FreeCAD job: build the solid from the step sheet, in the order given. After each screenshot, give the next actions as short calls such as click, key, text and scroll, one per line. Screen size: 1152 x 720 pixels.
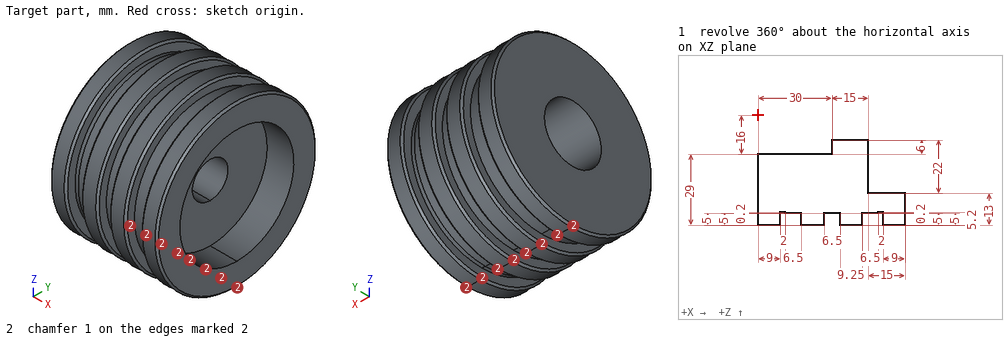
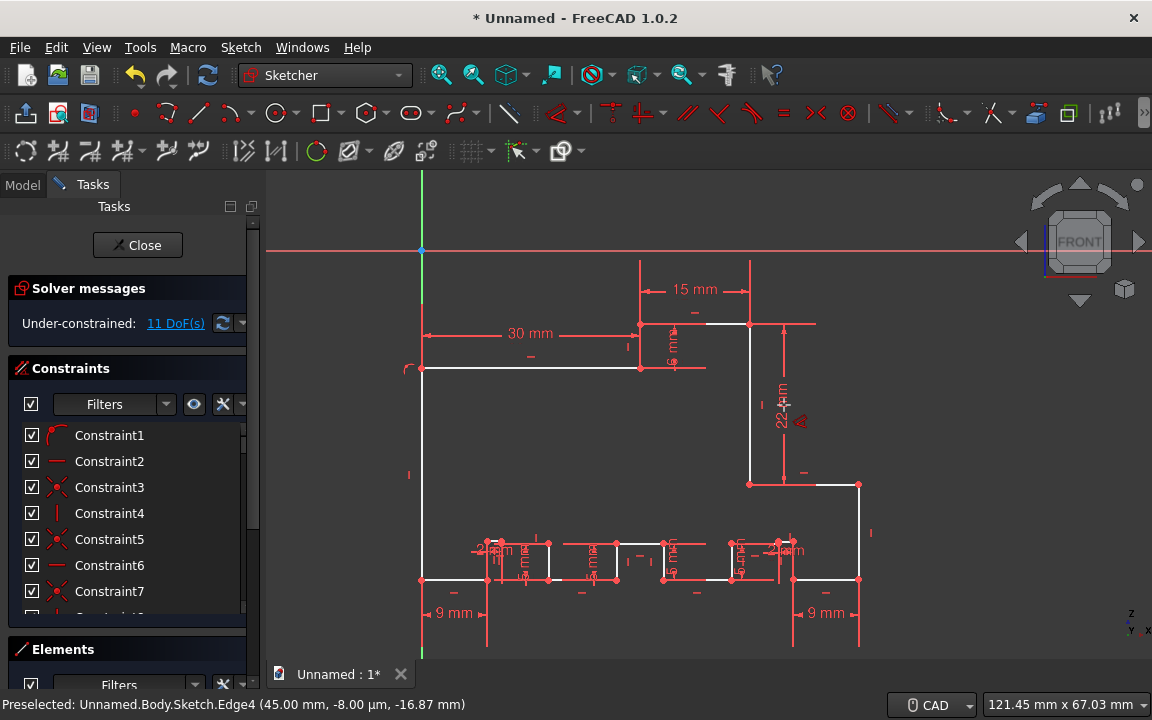
click(783, 485)
click(804, 519)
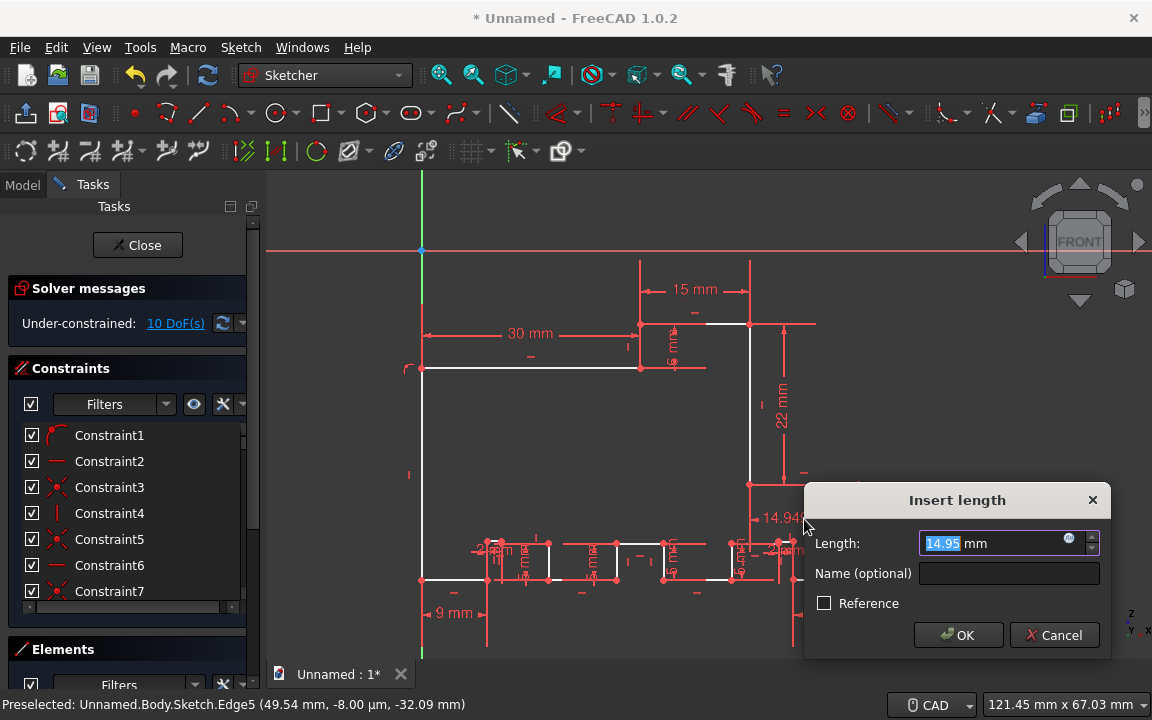
text(15)
key(Return)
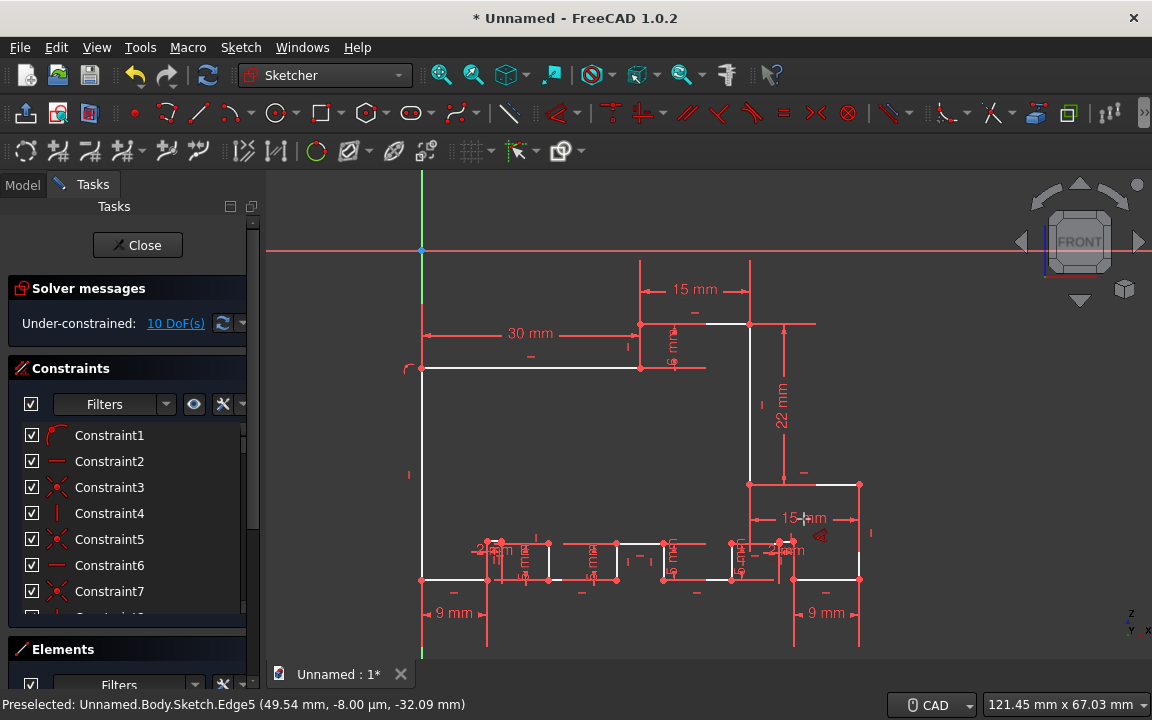
click(859, 513)
click(893, 532)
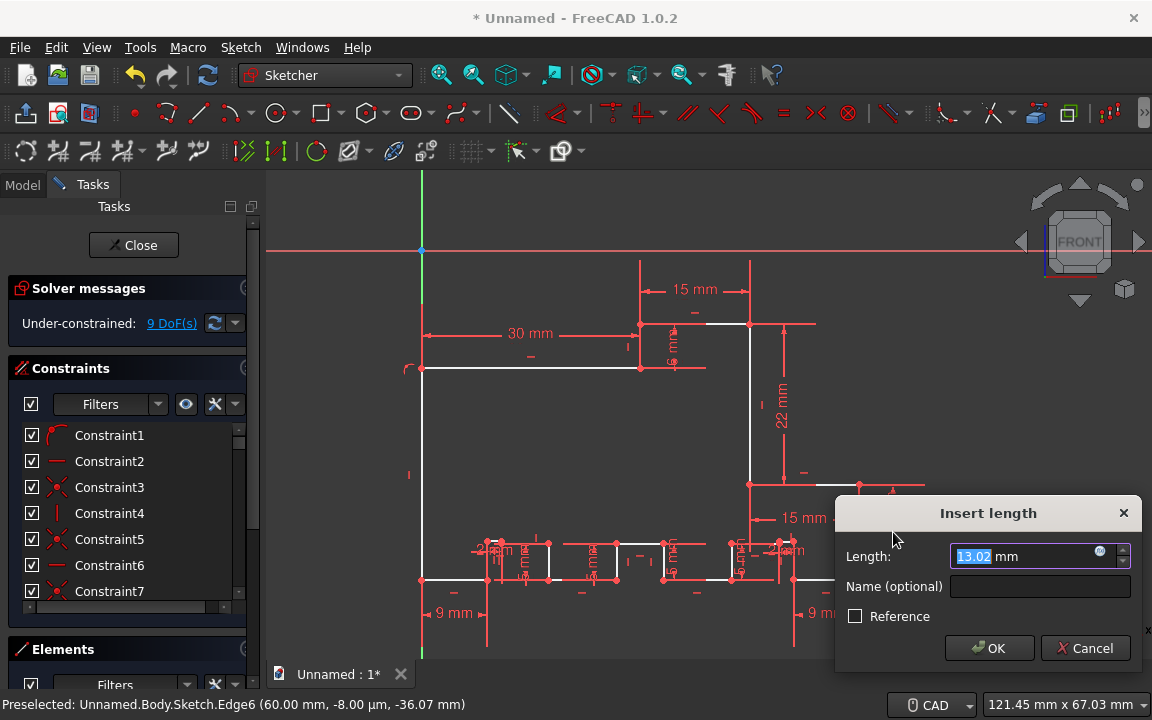
text(13)
key(Return)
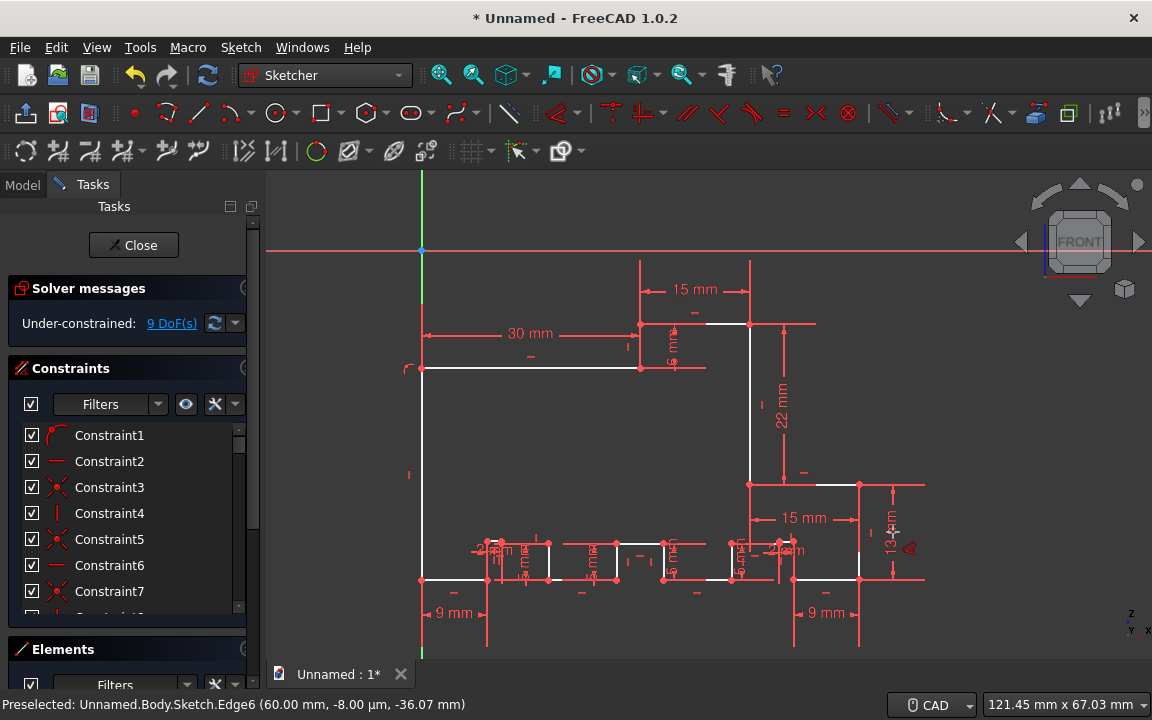
click(422, 517)
click(388, 474)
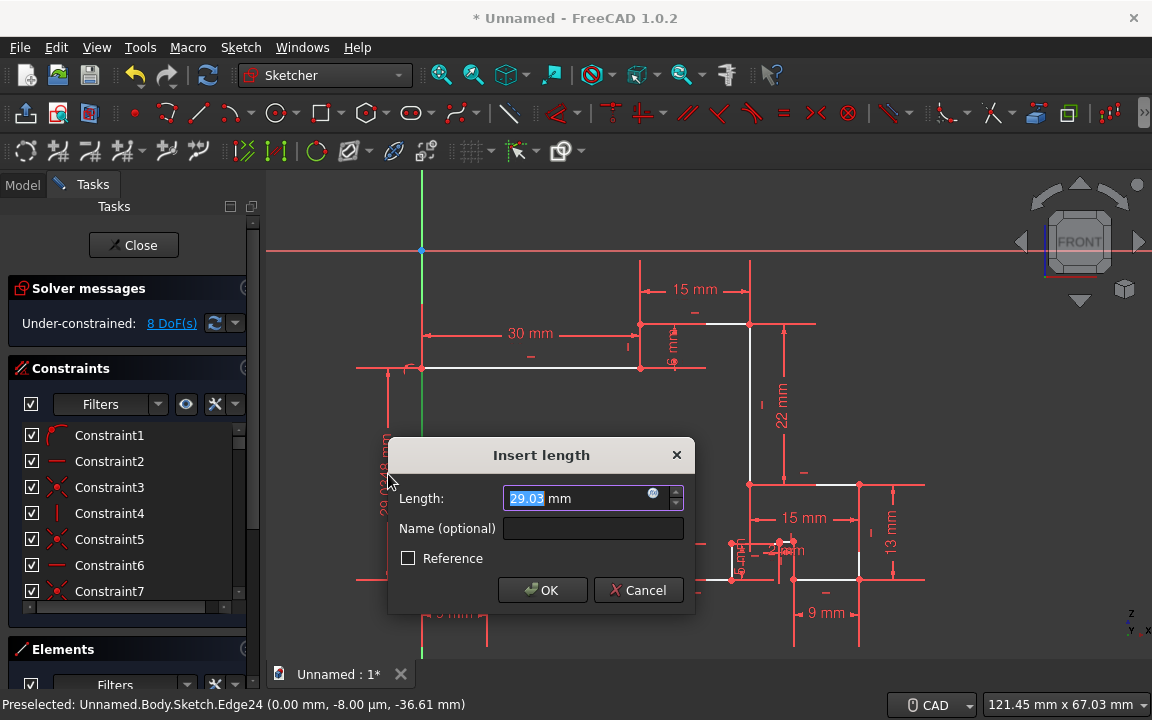
text(29)
key(Return)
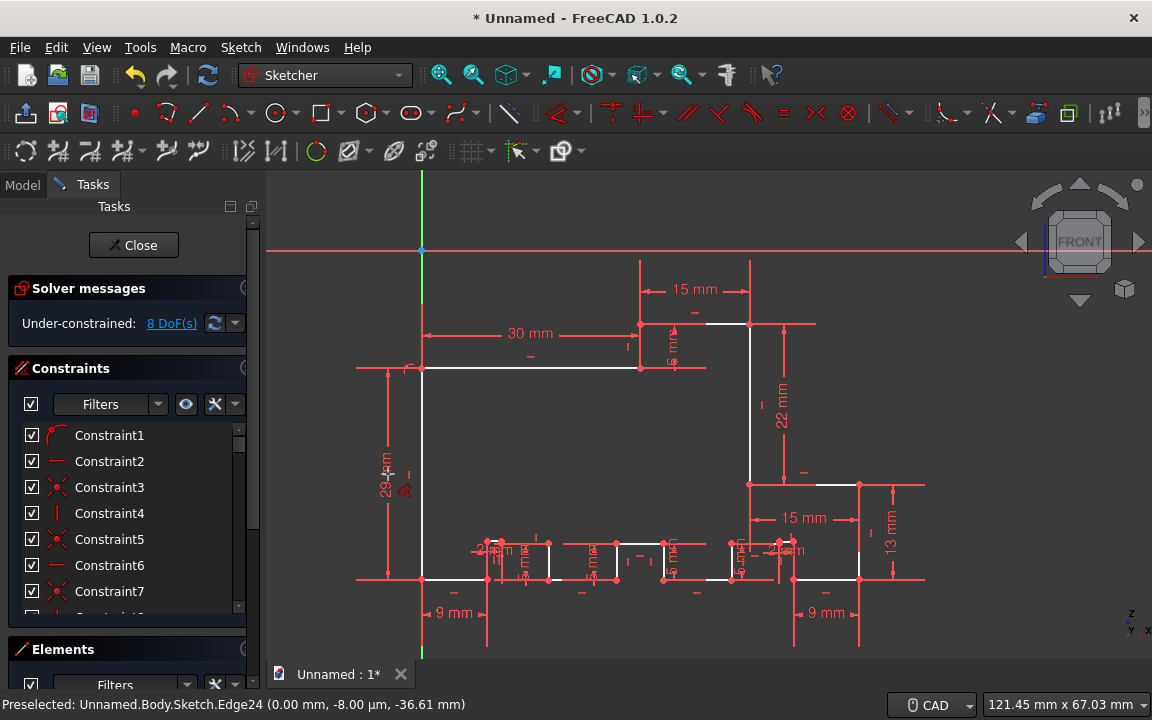
click(794, 568)
click(876, 561)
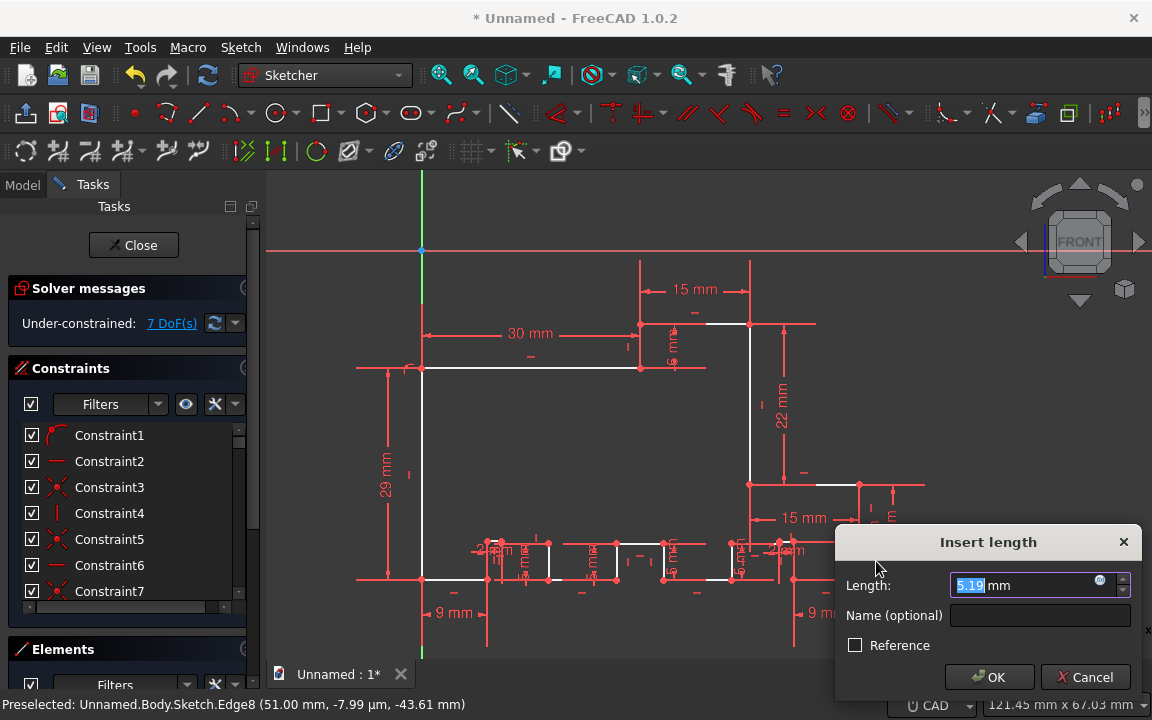
text(5.2)
key(Return)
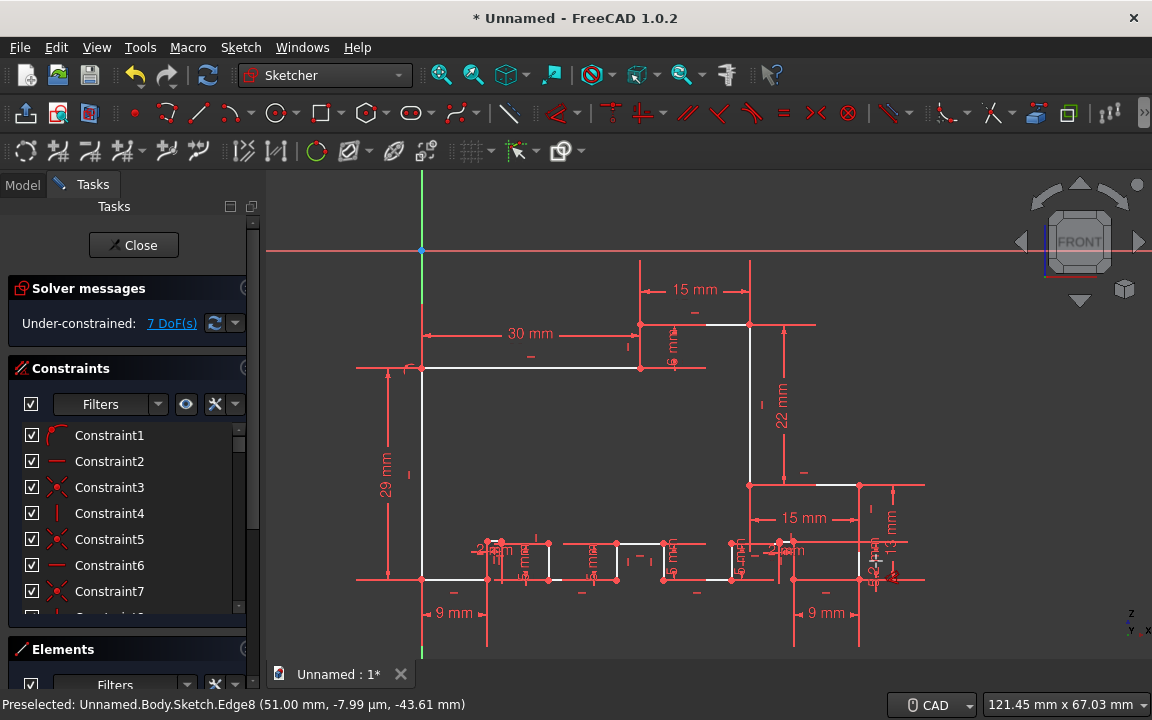
scroll(779, 543, up, 17)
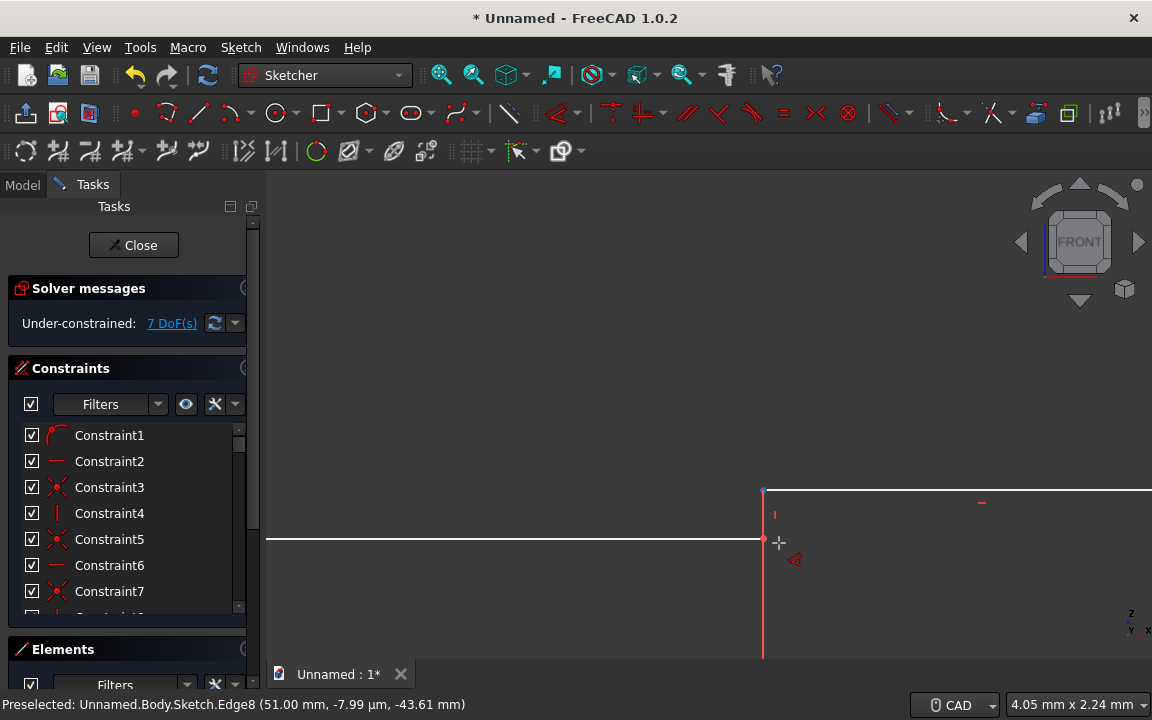
click(763, 515)
click(797, 515)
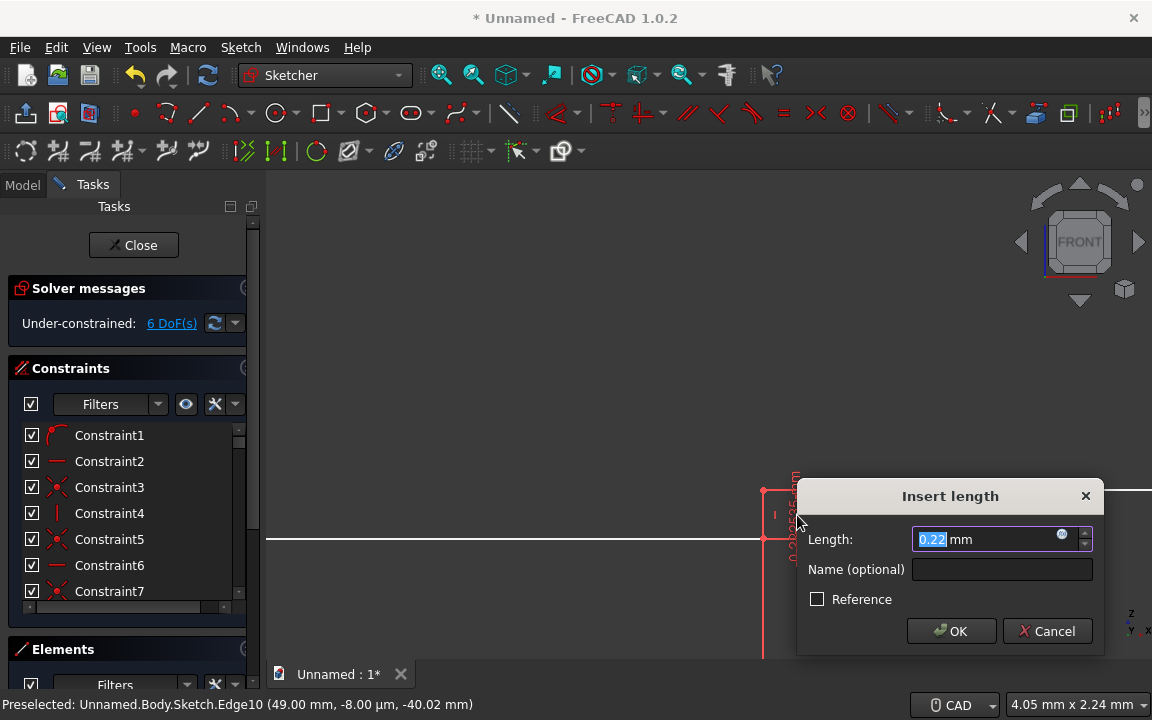
text(0.2)
key(Return)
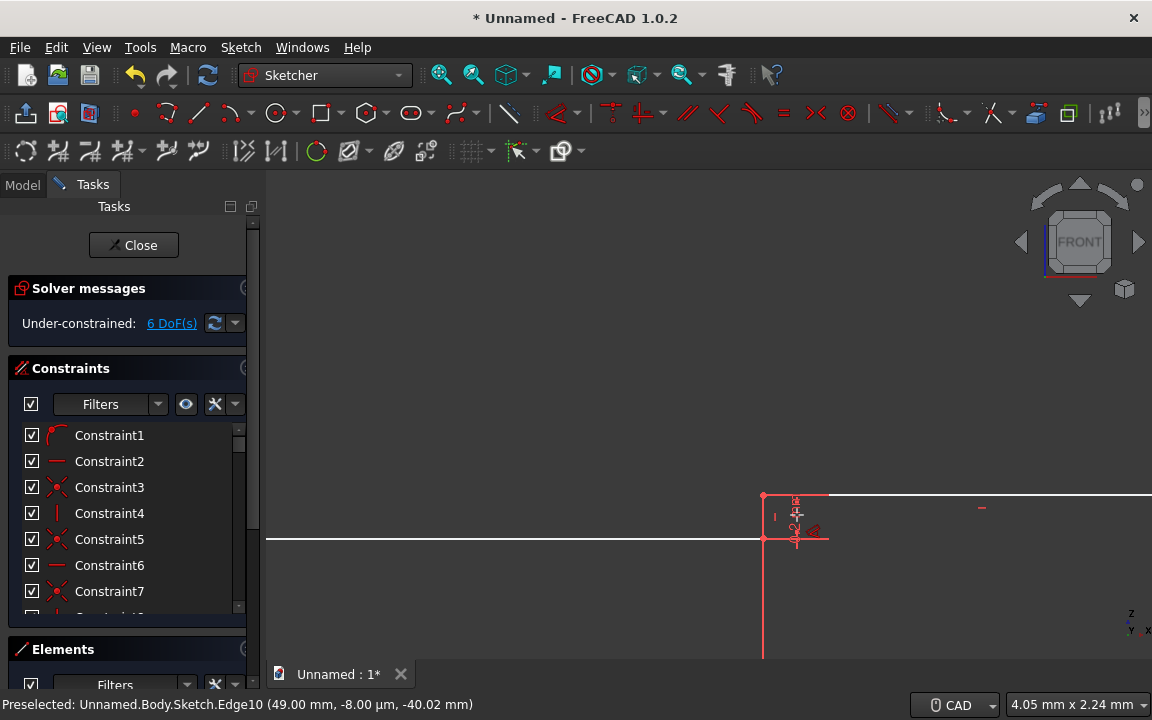
scroll(780, 543, down, 17)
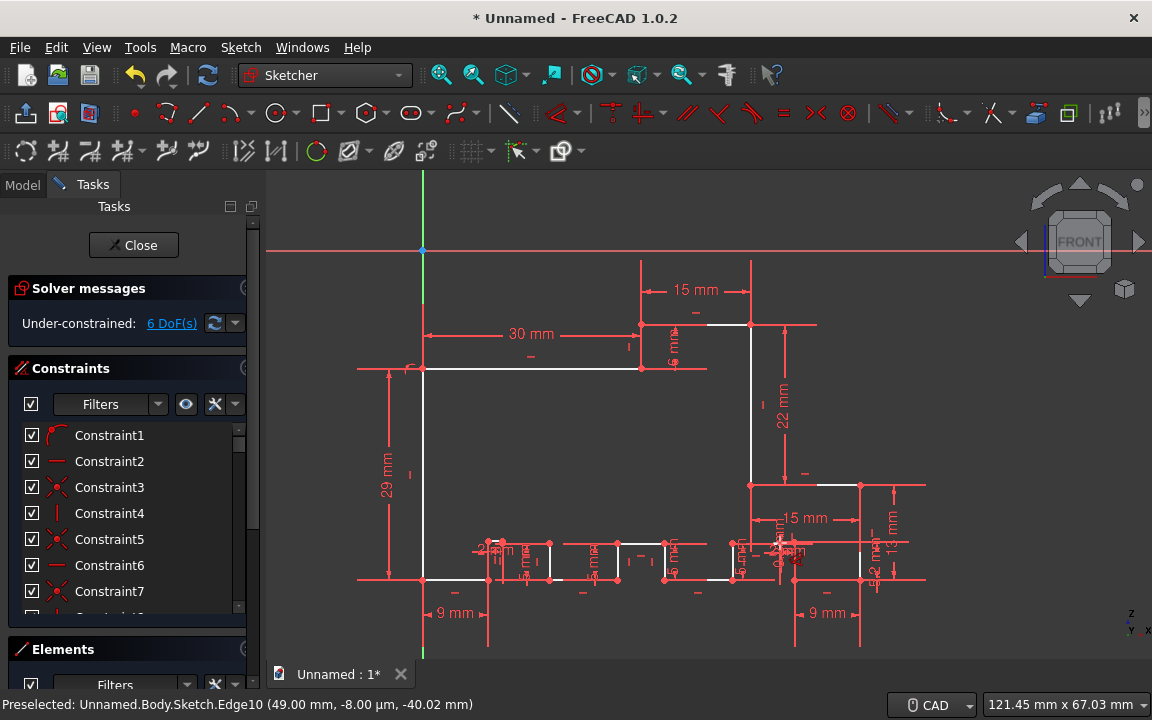
click(766, 544)
click(756, 578)